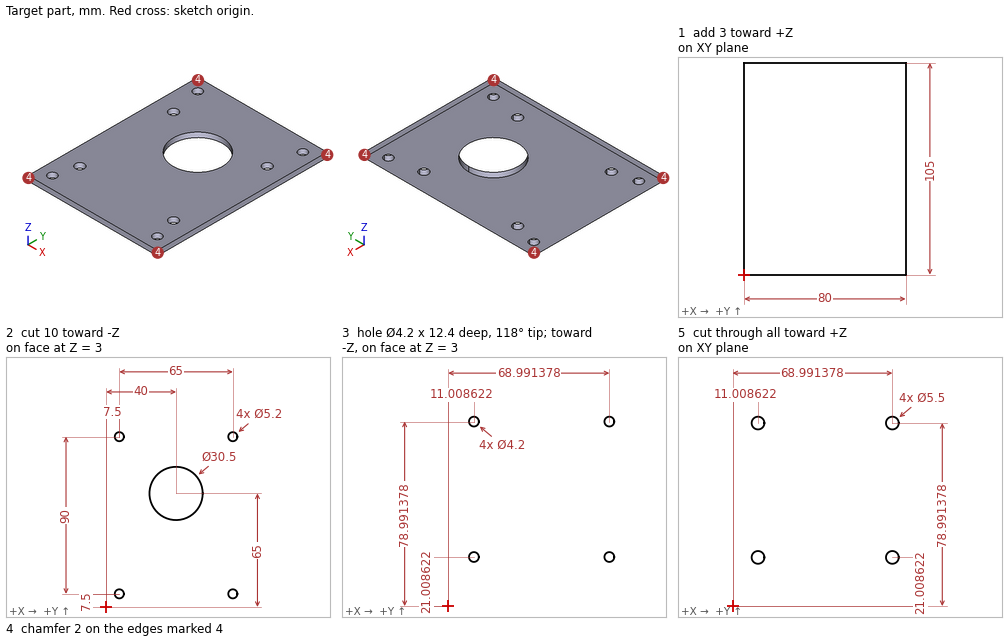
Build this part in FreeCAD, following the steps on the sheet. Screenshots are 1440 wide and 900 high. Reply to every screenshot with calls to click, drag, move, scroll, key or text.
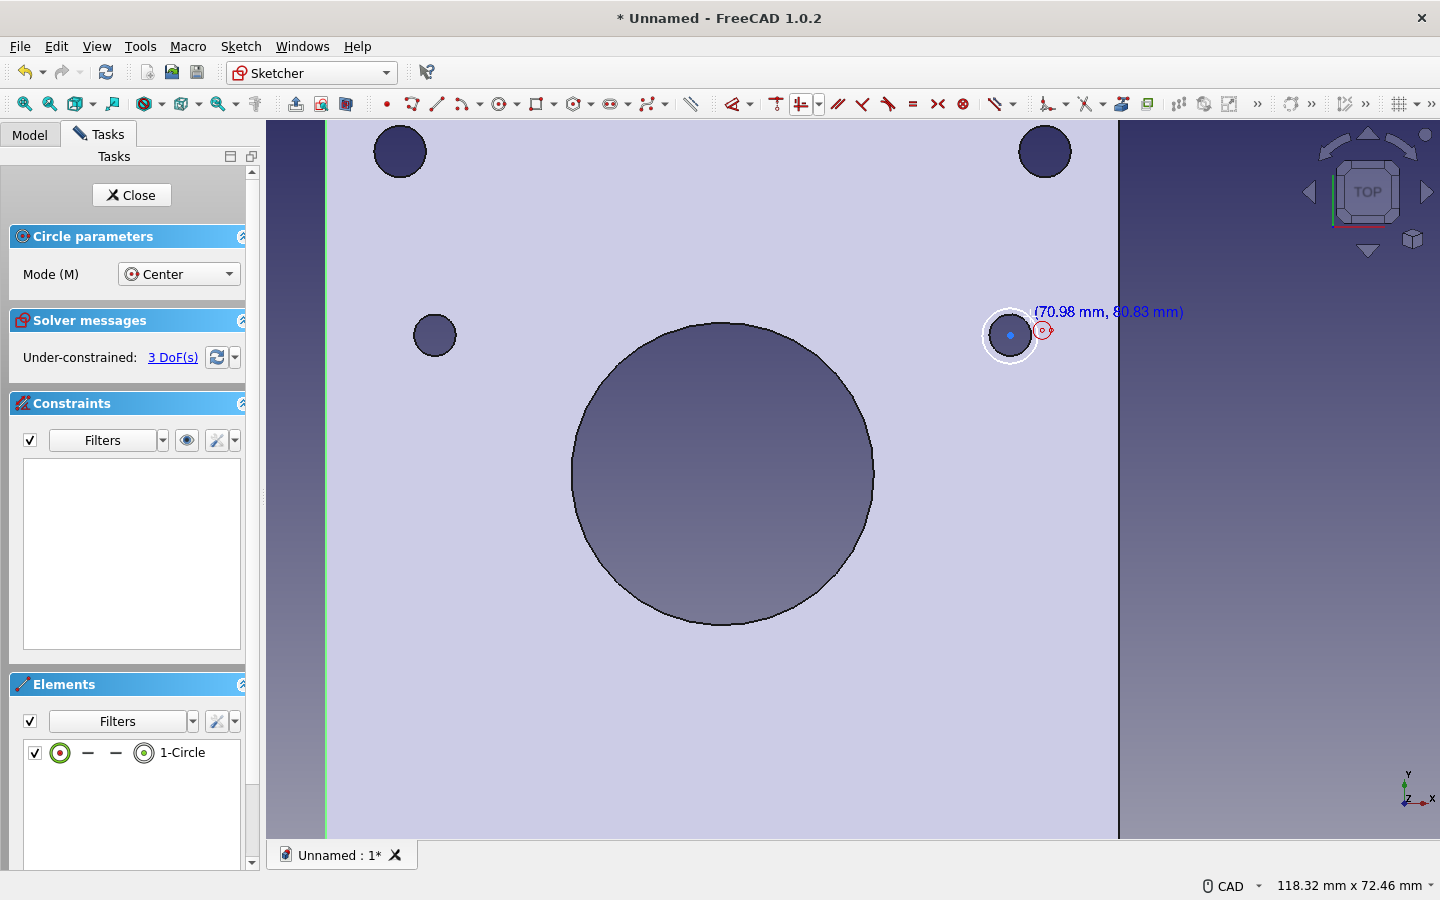
click(435, 335)
click(454, 316)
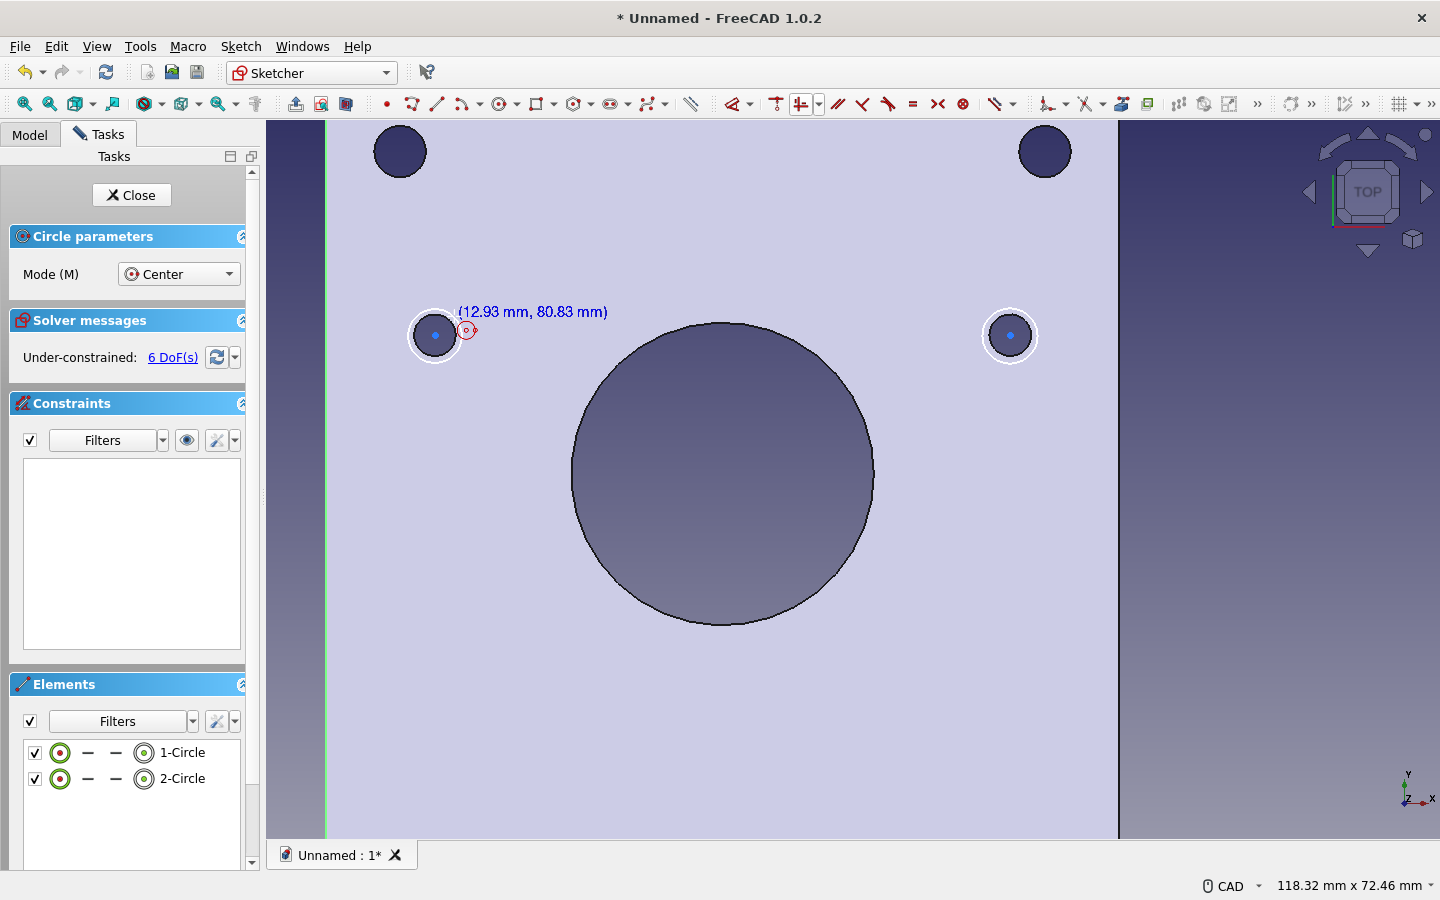
scroll(910, 195, down, 3)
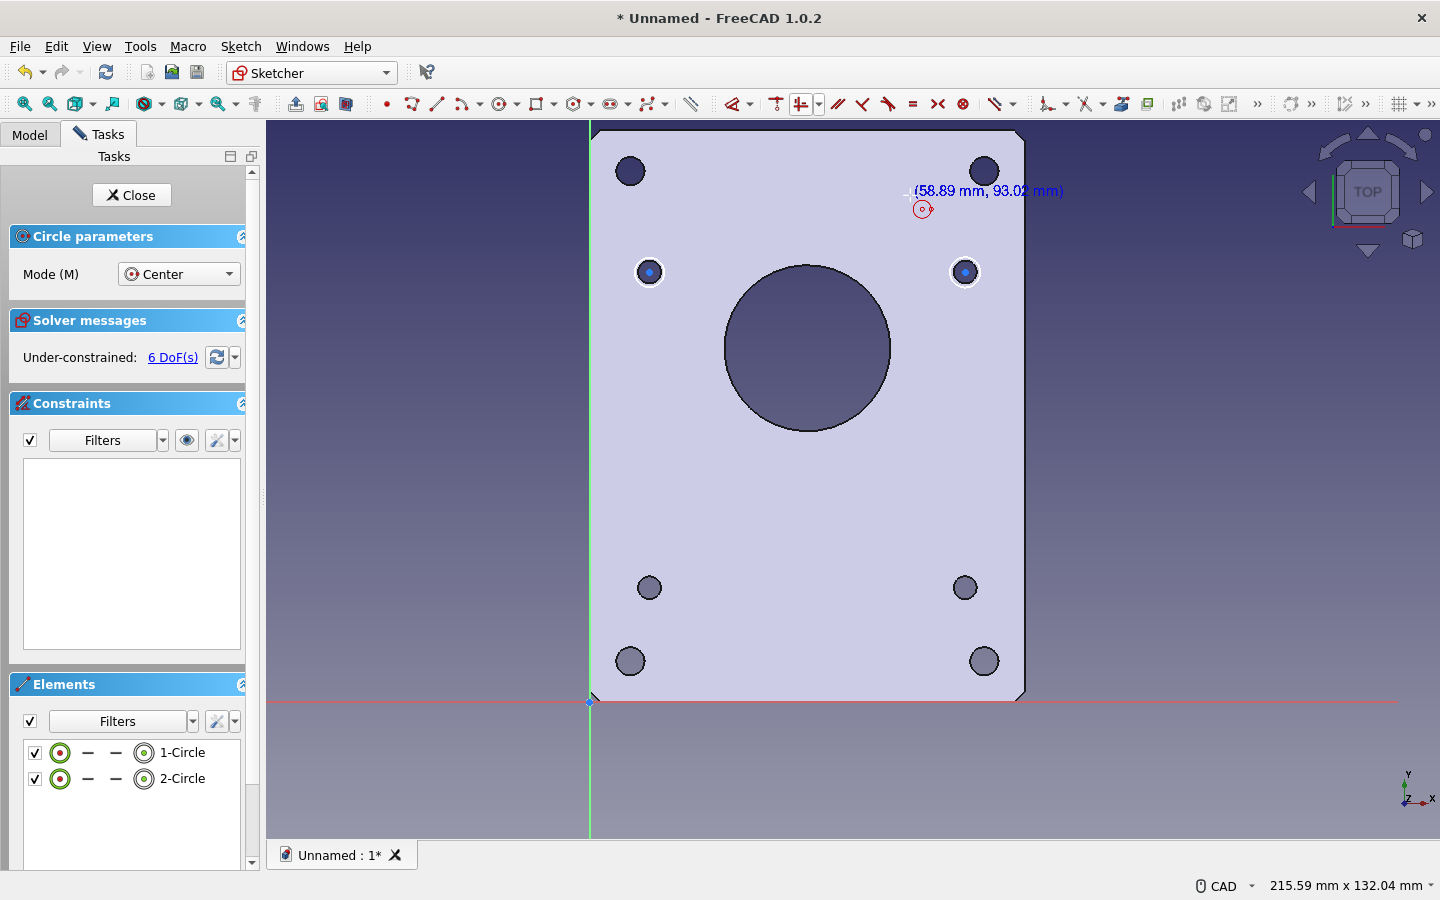
scroll(965, 588, up, 3)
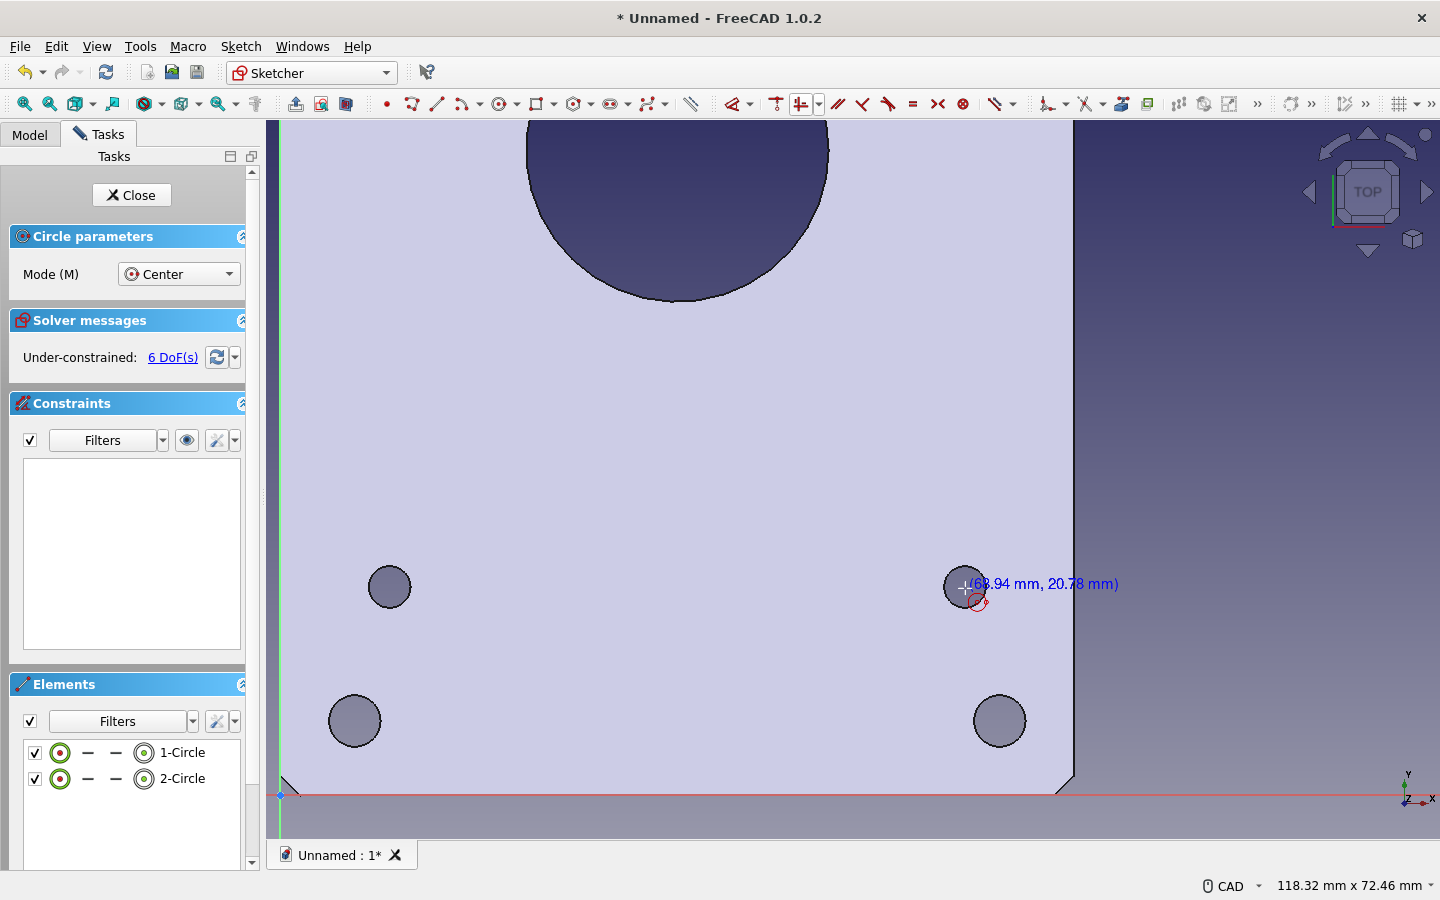
click(965, 587)
click(984, 568)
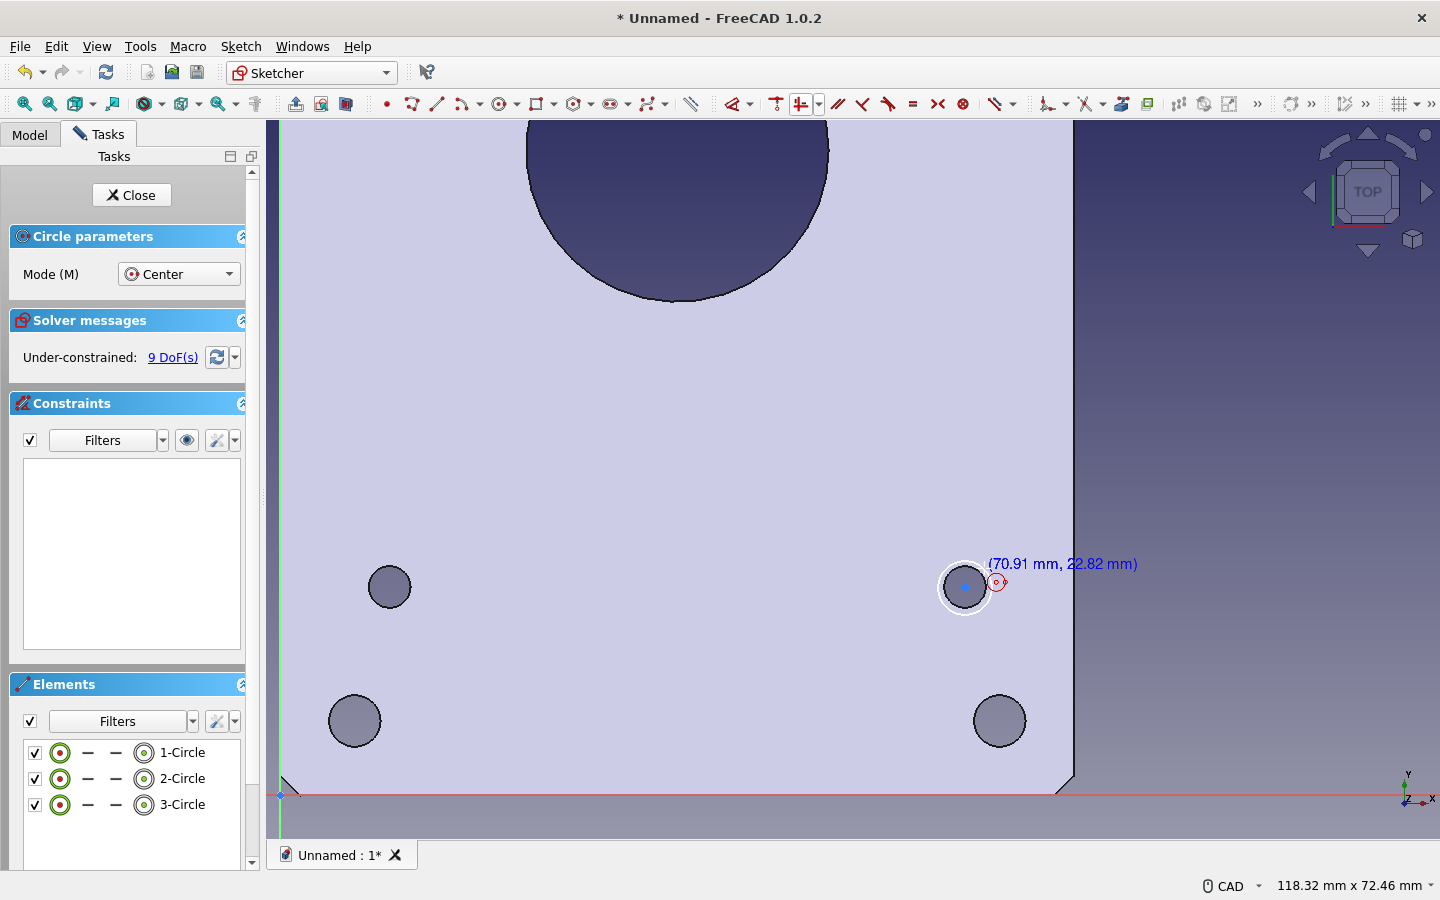
click(390, 587)
click(409, 568)
key(Escape)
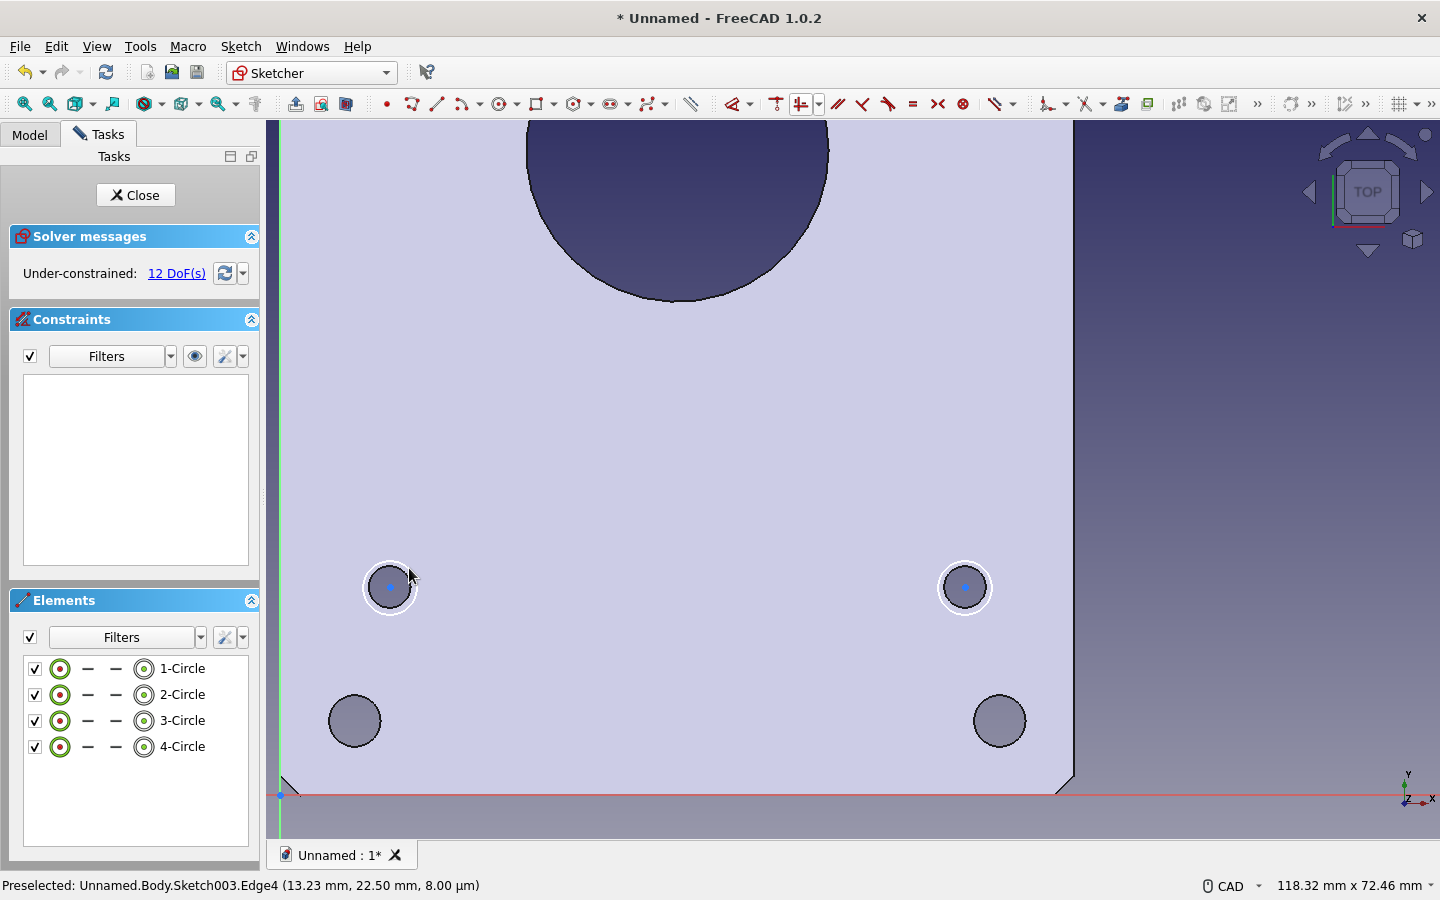
scroll(965, 588, down, 3)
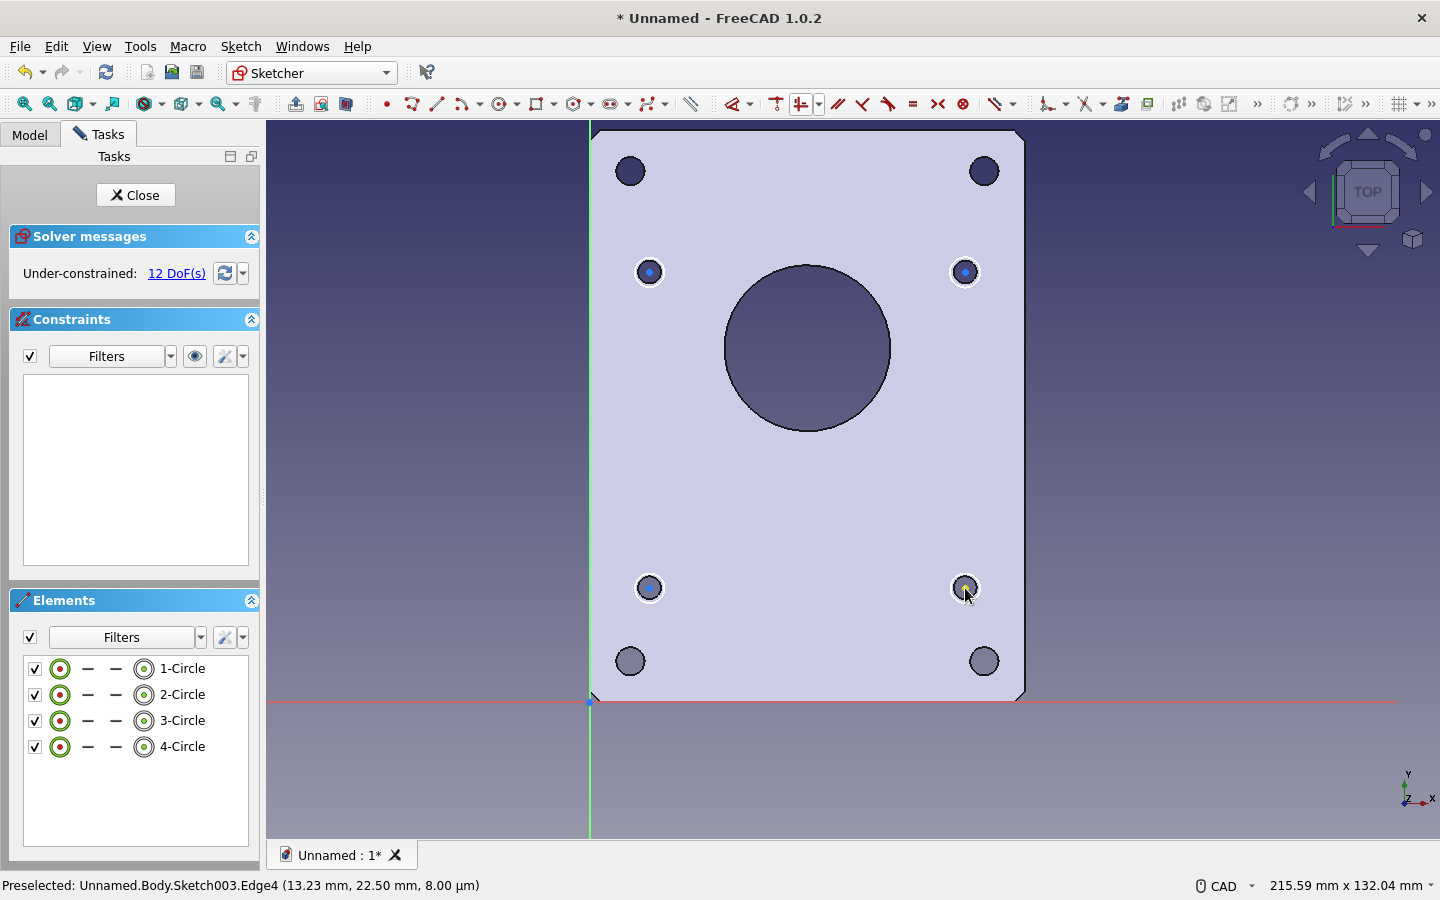
click(976, 262)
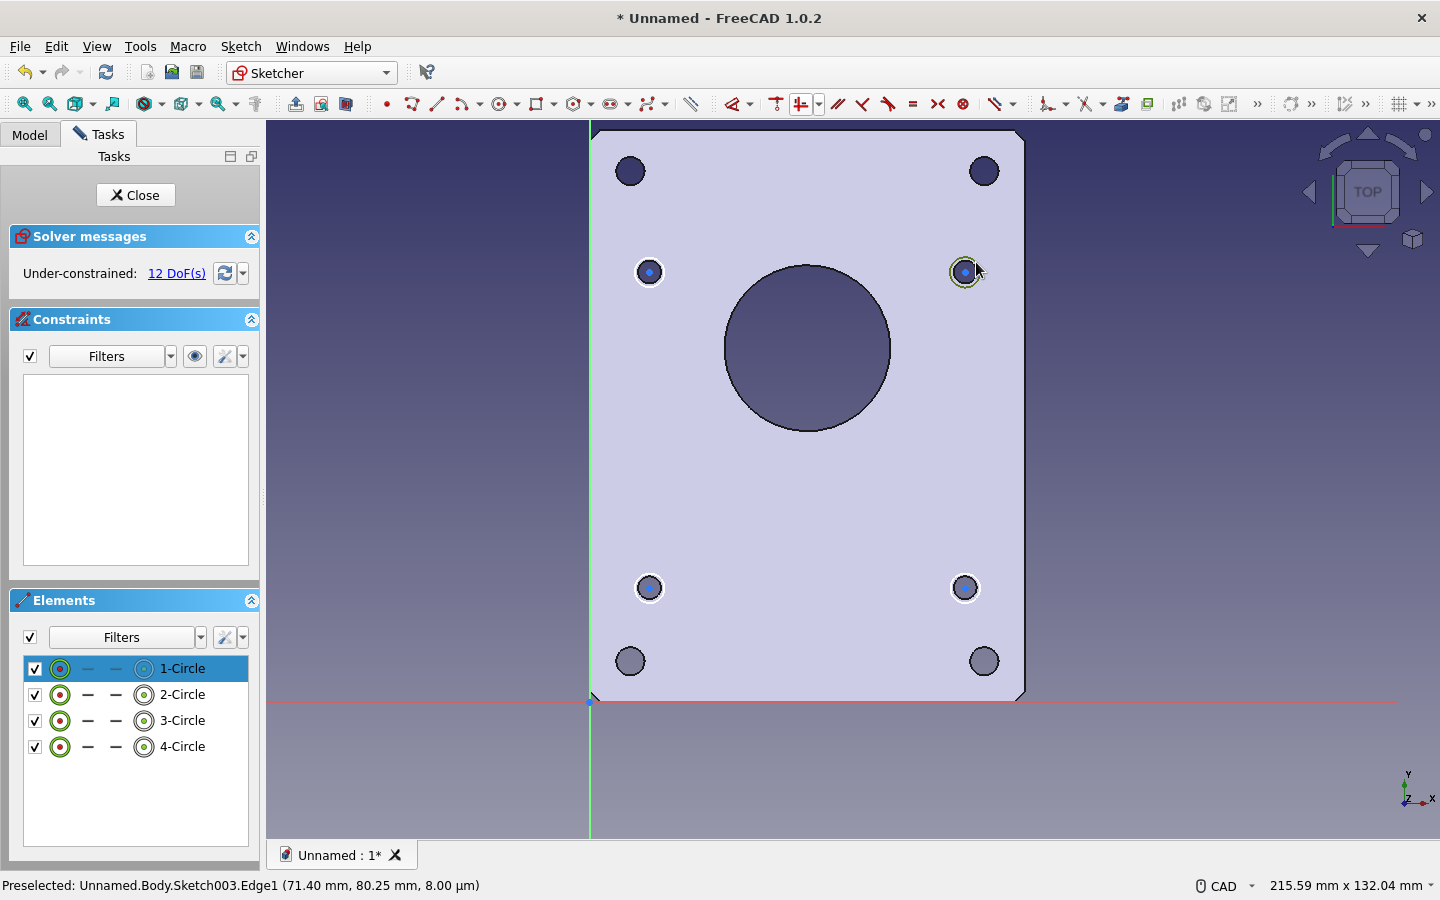
click(660, 262)